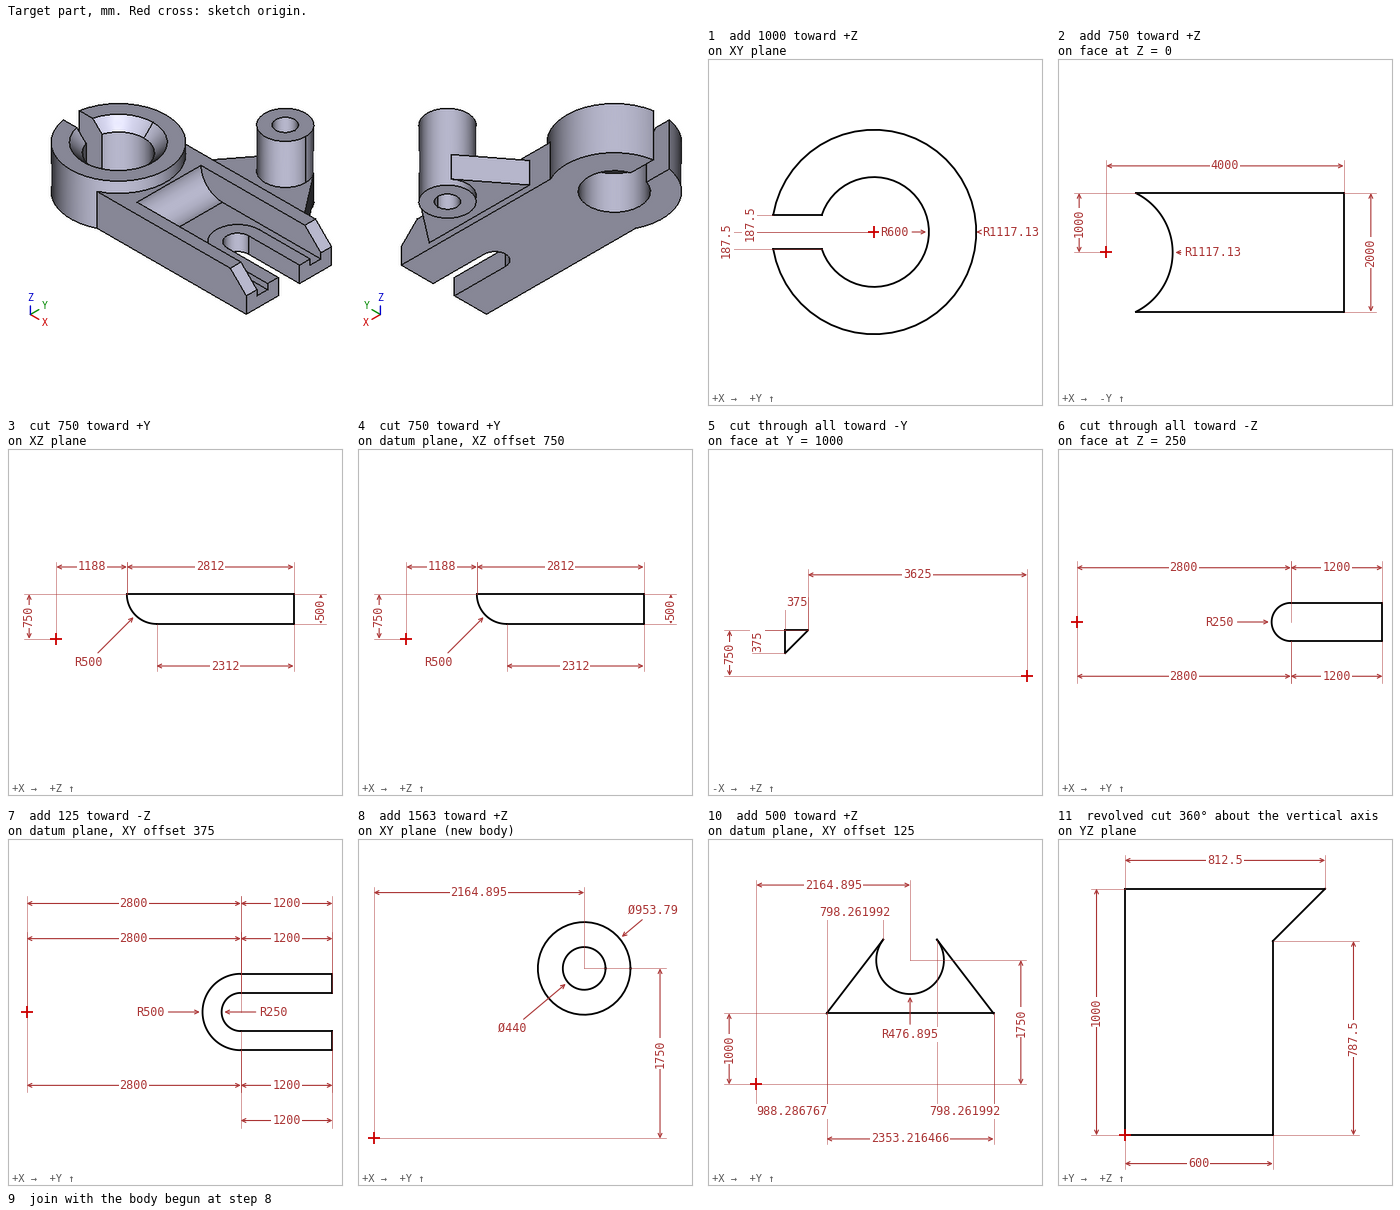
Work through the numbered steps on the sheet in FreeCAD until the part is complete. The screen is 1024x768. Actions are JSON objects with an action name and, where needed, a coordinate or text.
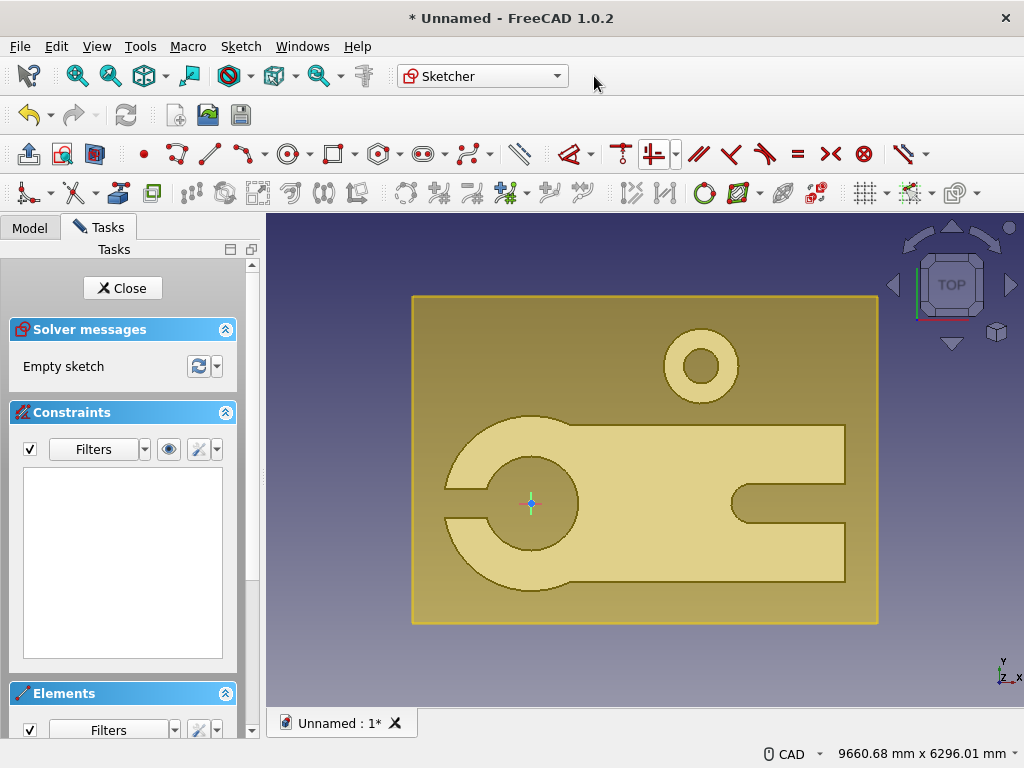
{"action": "scroll", "coordinate": [837, 349], "scroll_direction": "up", "scroll_amount": 2}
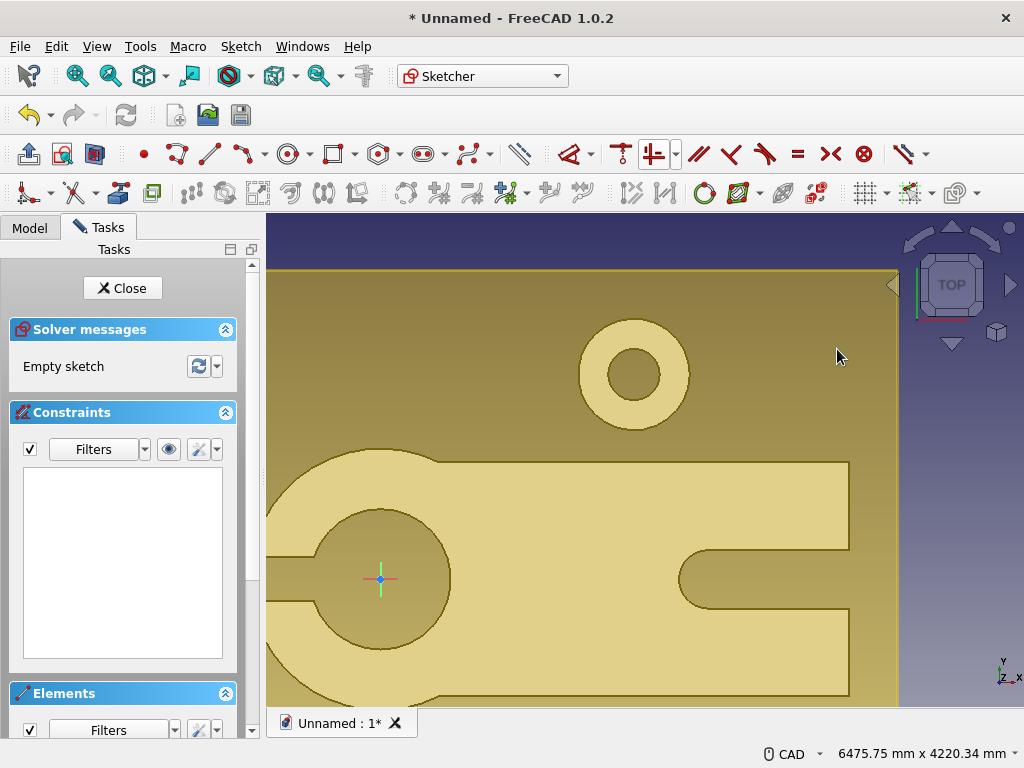
{"action": "key", "text": "g m"}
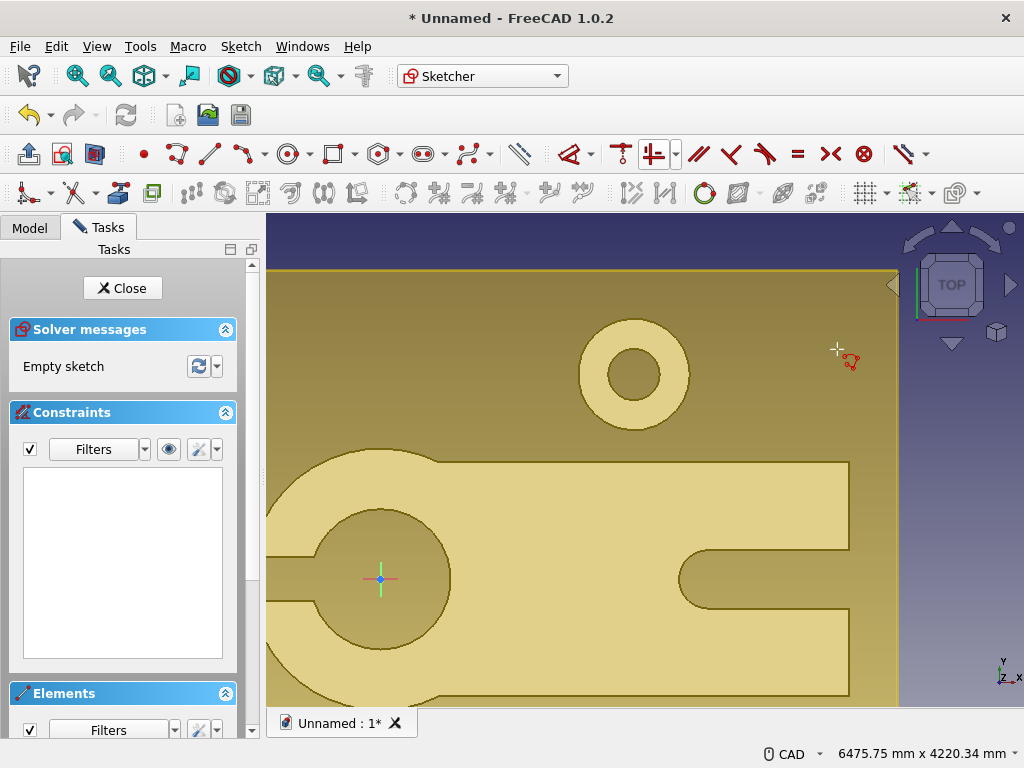
{"action": "left_click", "coordinate": [590, 341]}
{"action": "left_click", "coordinate": [496, 462]}
{"action": "left_click", "coordinate": [772, 462]}
{"action": "left_click", "coordinate": [678, 341]}
{"action": "right_click", "coordinate": [678, 341]}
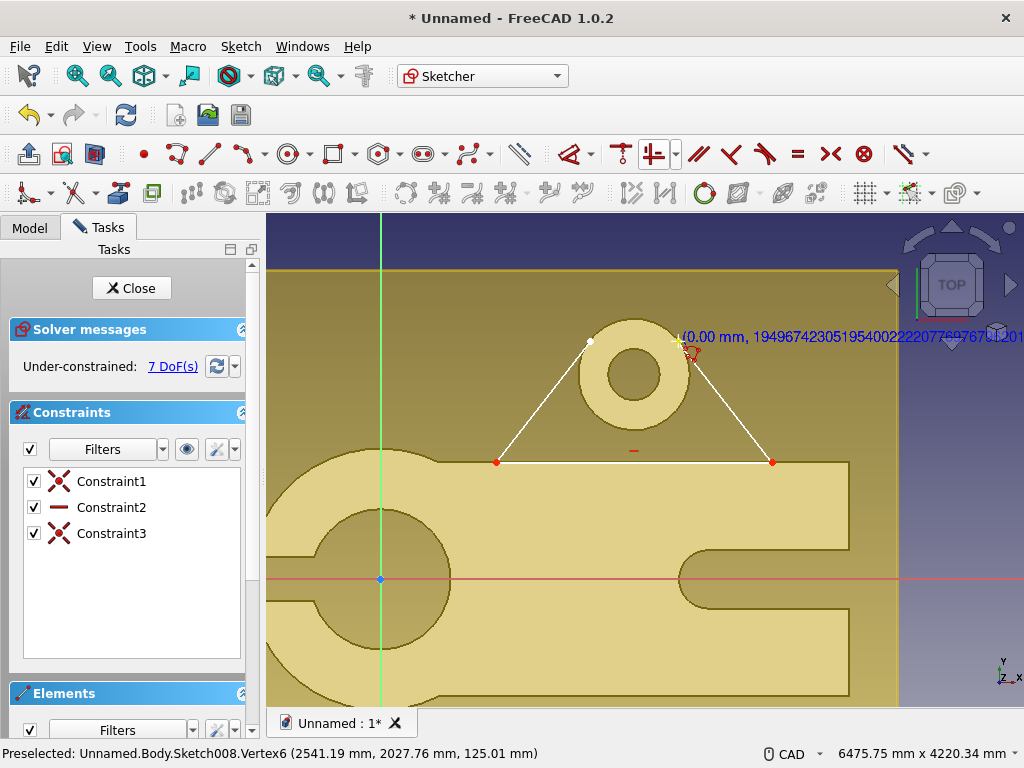
{"action": "key", "text": "g 3 a"}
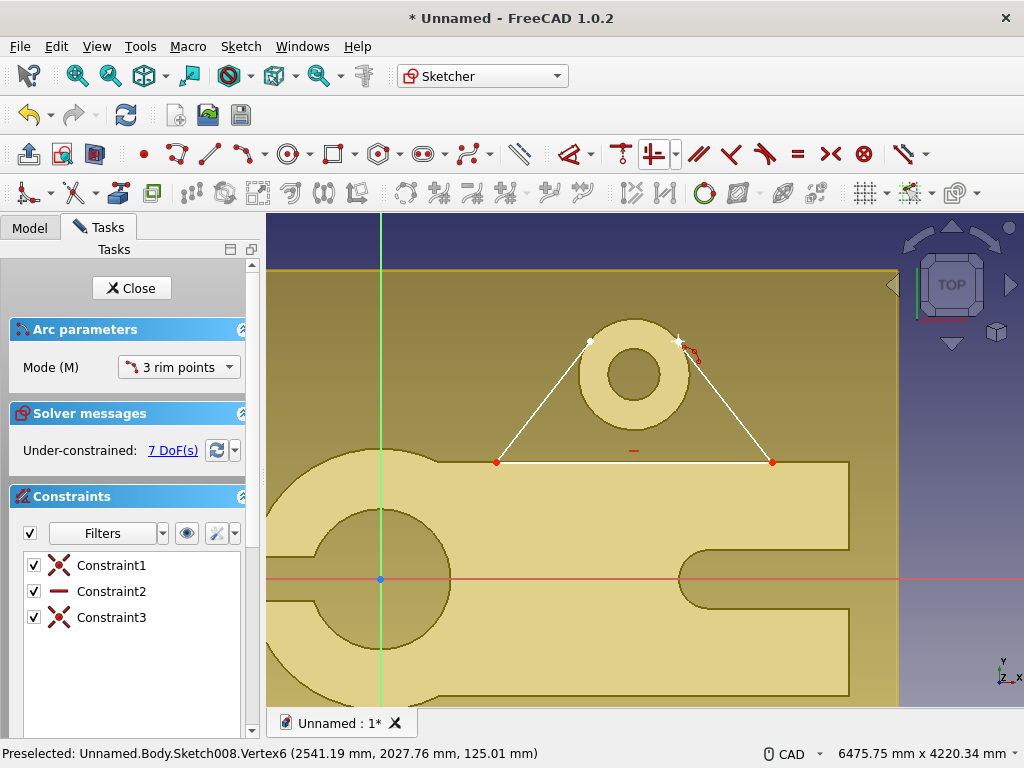
{"action": "left_click", "coordinate": [678, 342]}
{"action": "left_click", "coordinate": [590, 342]}
{"action": "left_click", "coordinate": [634, 430]}
{"action": "key", "text": "Escape"}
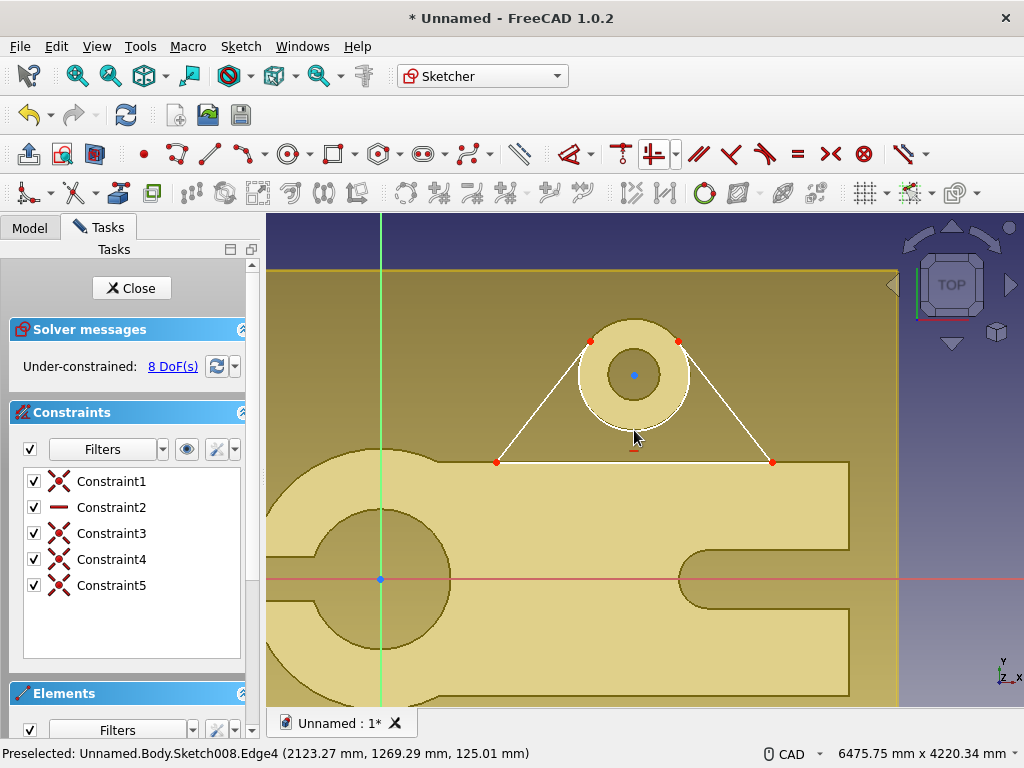
{"action": "key", "text": "d"}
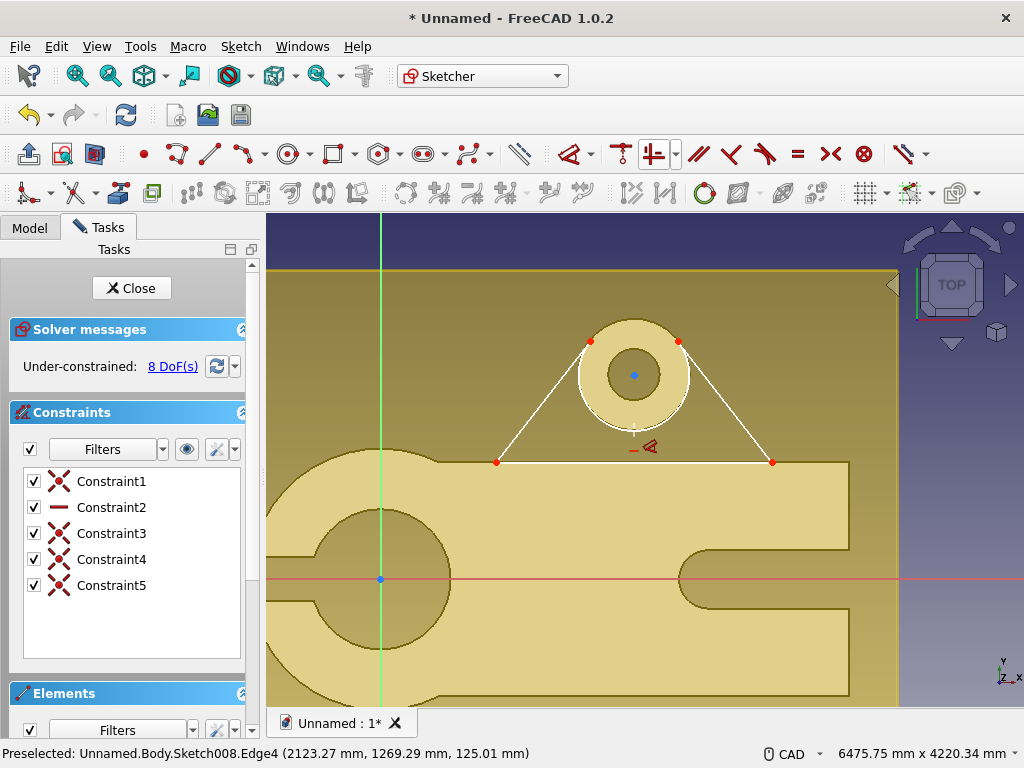
{"action": "left_click", "coordinate": [591, 411]}
{"action": "left_click", "coordinate": [566, 431]}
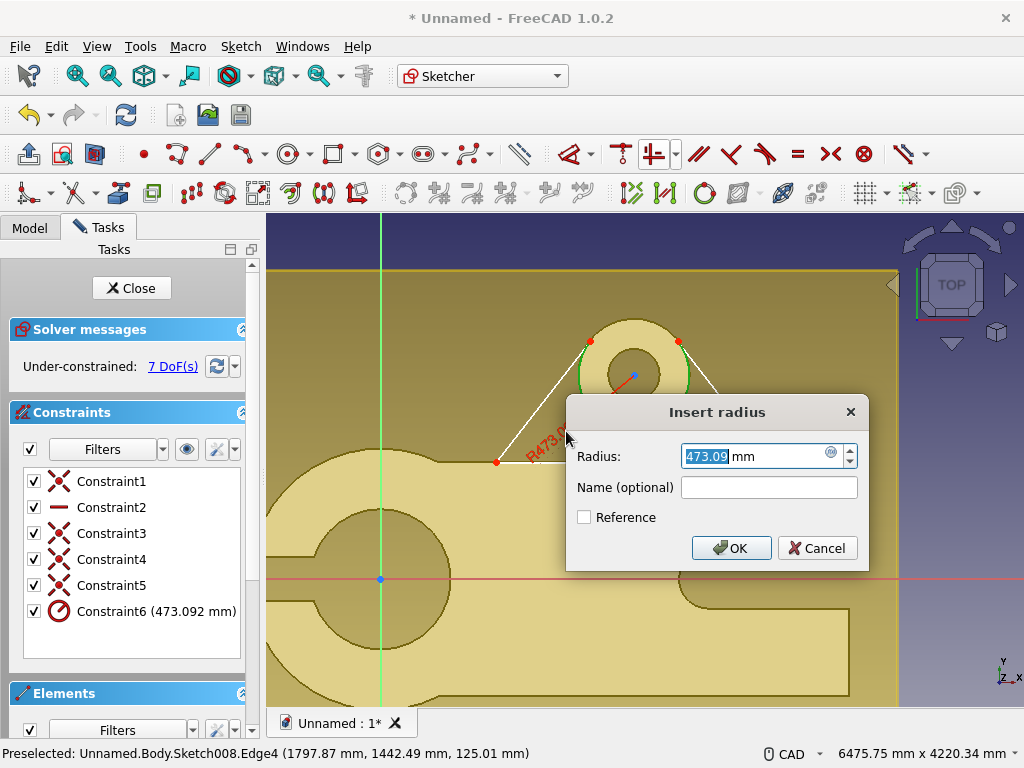
{"action": "type", "text": "476.895"}
{"action": "key", "text": "Return"}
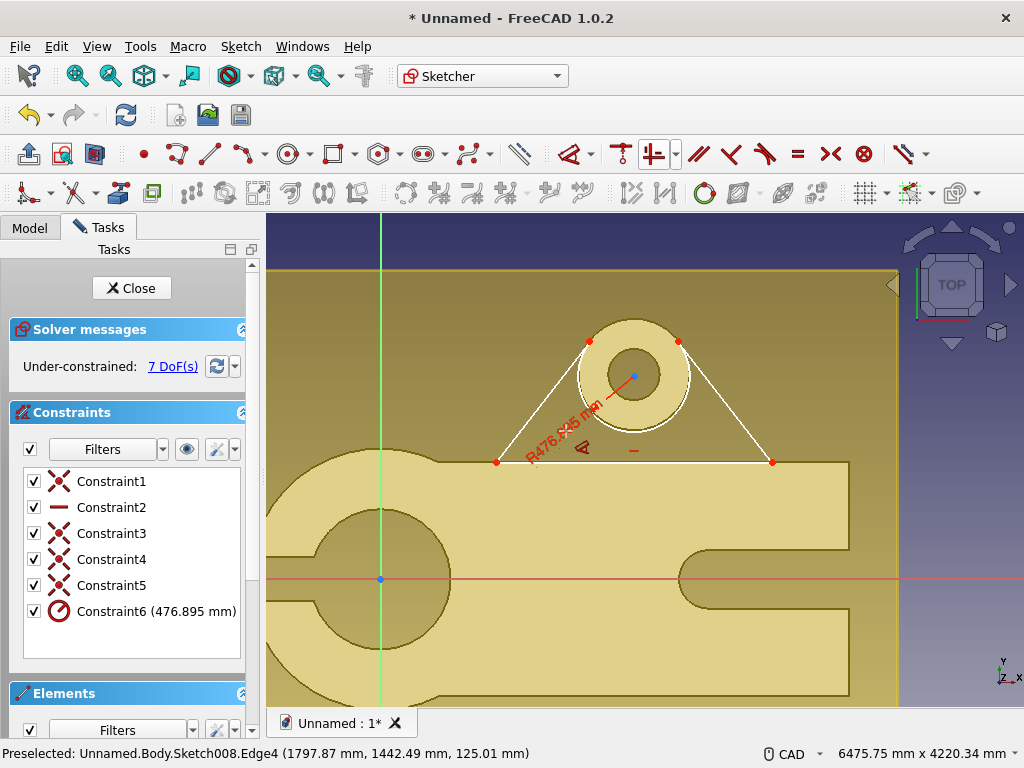
{"action": "left_click", "coordinate": [496, 463]}
{"action": "left_click", "coordinate": [347, 521]}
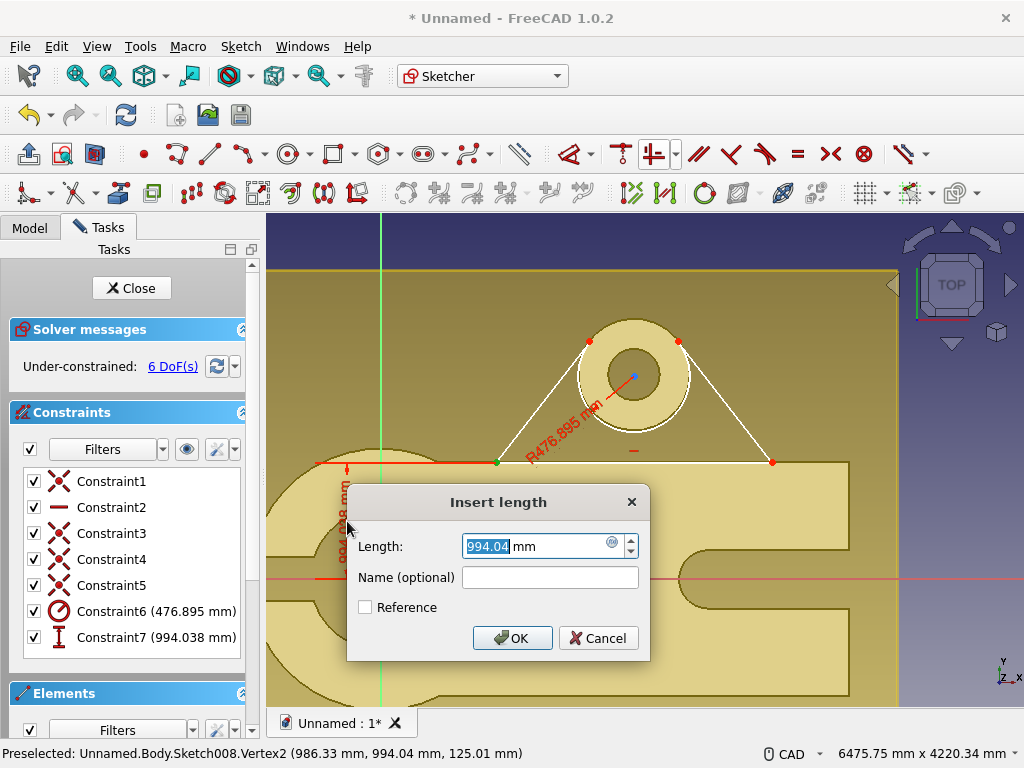
{"action": "type", "text": "1000"}
{"action": "key", "text": "Return"}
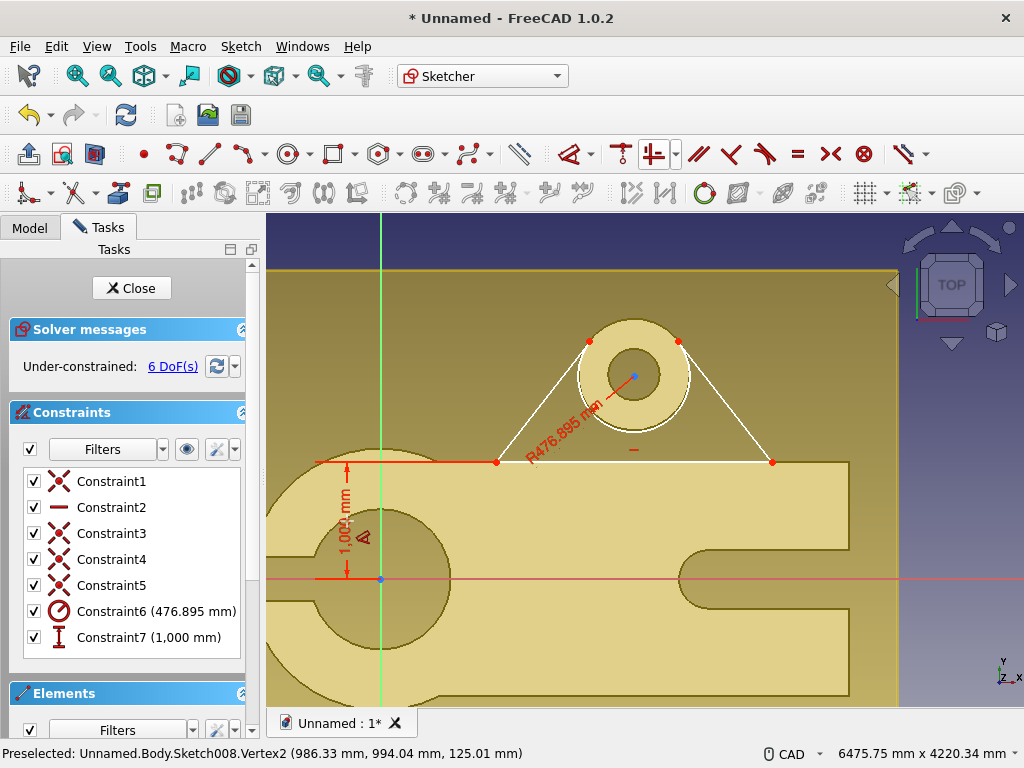
{"action": "left_click", "coordinate": [634, 376]}
{"action": "left_click", "coordinate": [347, 478]}